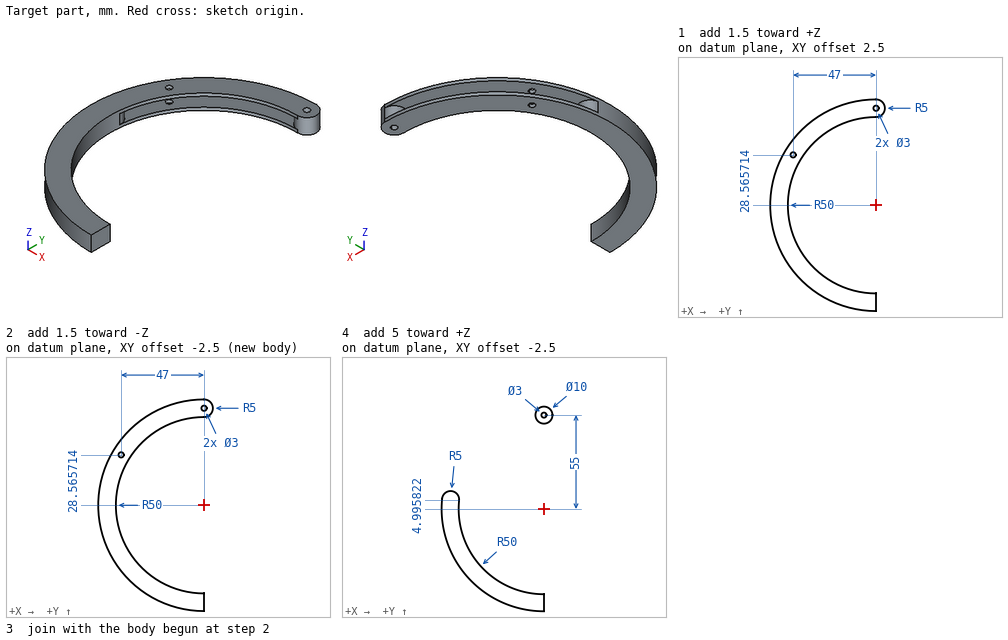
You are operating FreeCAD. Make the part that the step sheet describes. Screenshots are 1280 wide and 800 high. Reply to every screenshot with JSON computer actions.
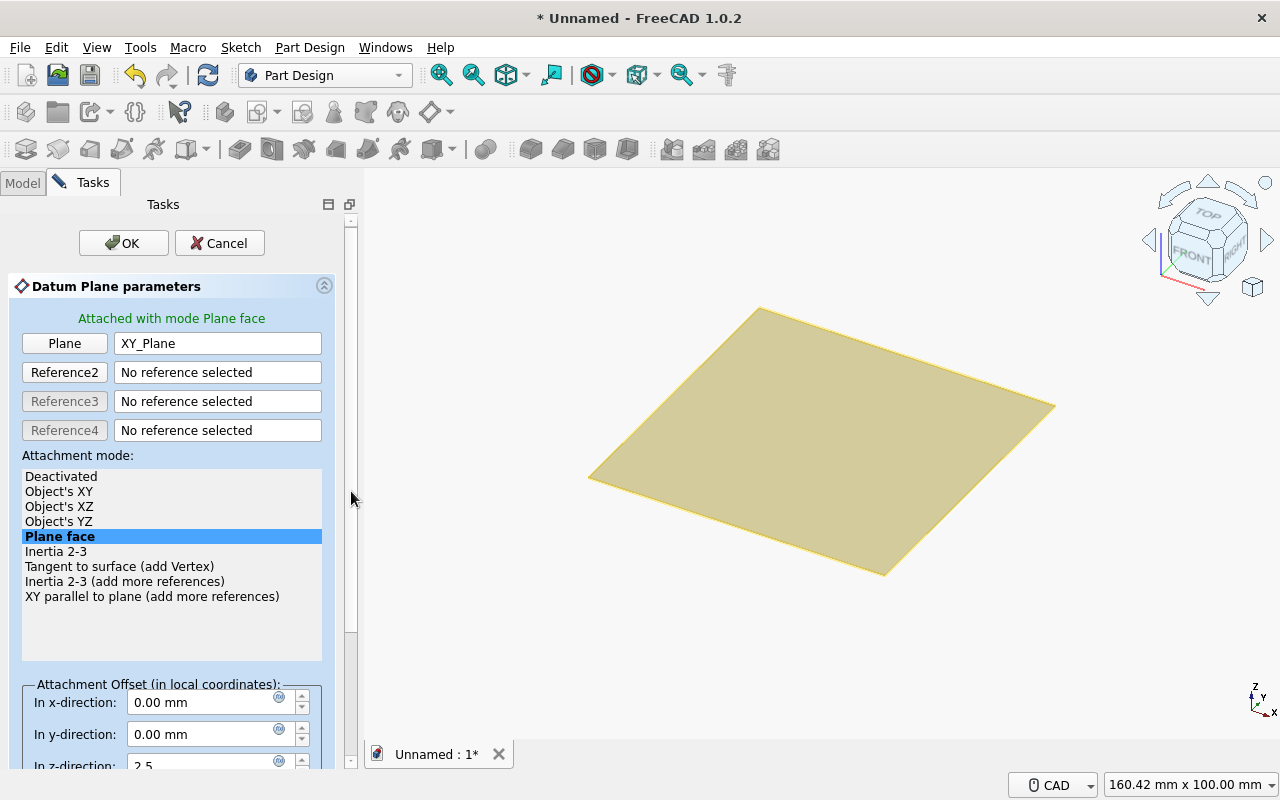
{"action": "left_click", "coordinate": [124, 243]}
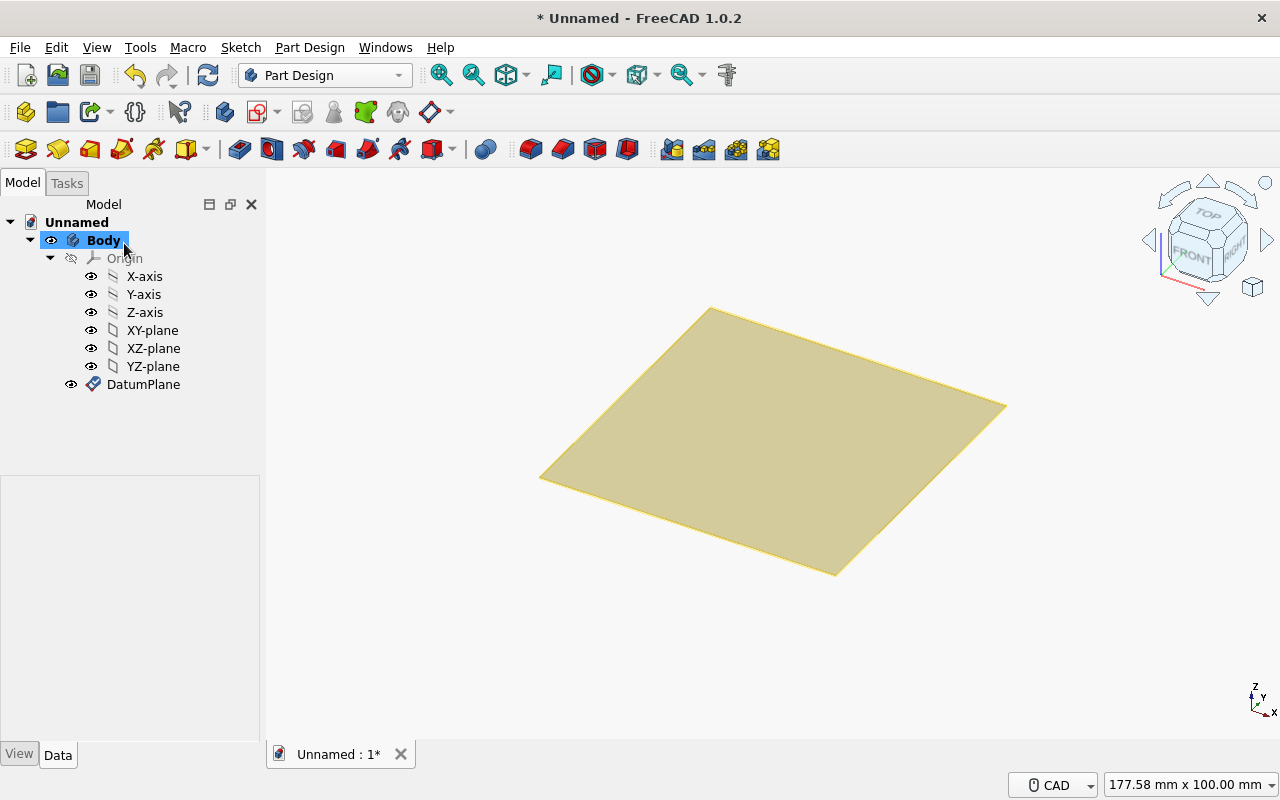
{"action": "left_click", "coordinate": [116, 384]}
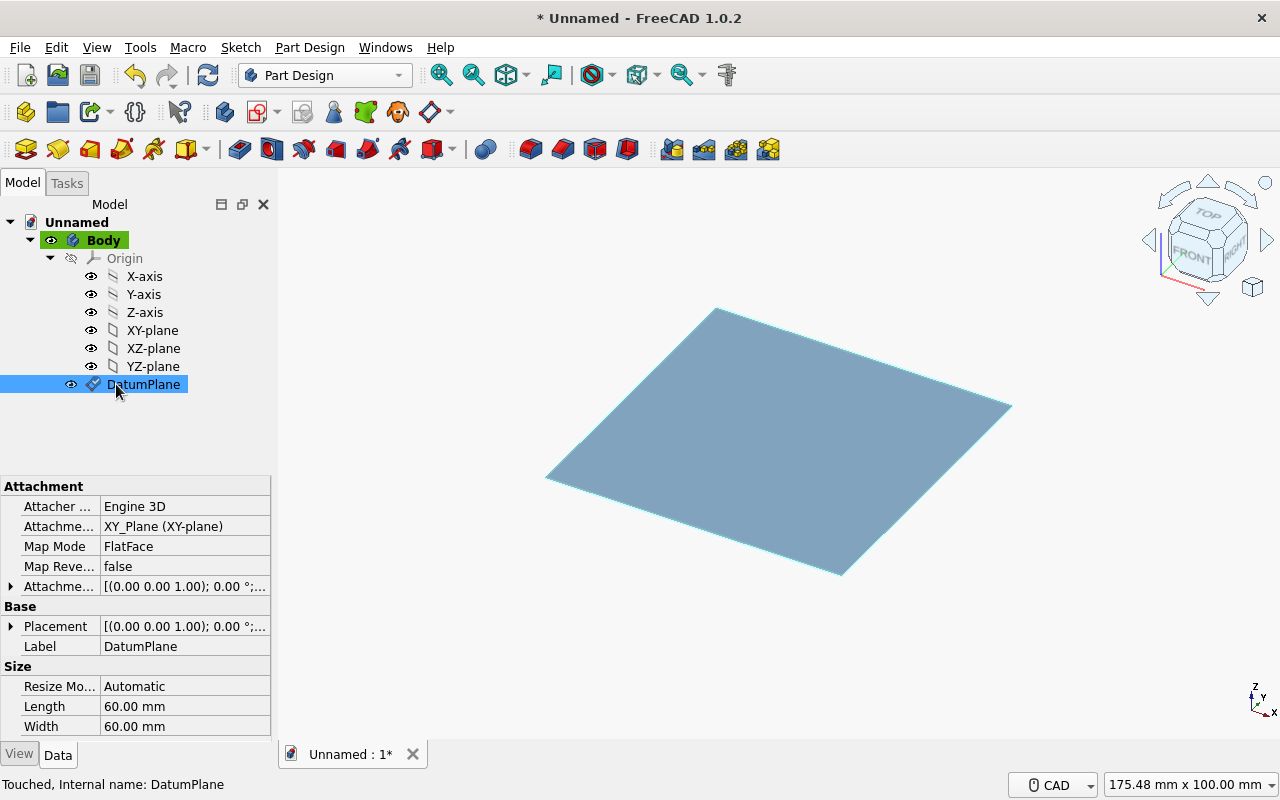
{"action": "left_click", "coordinate": [258, 112]}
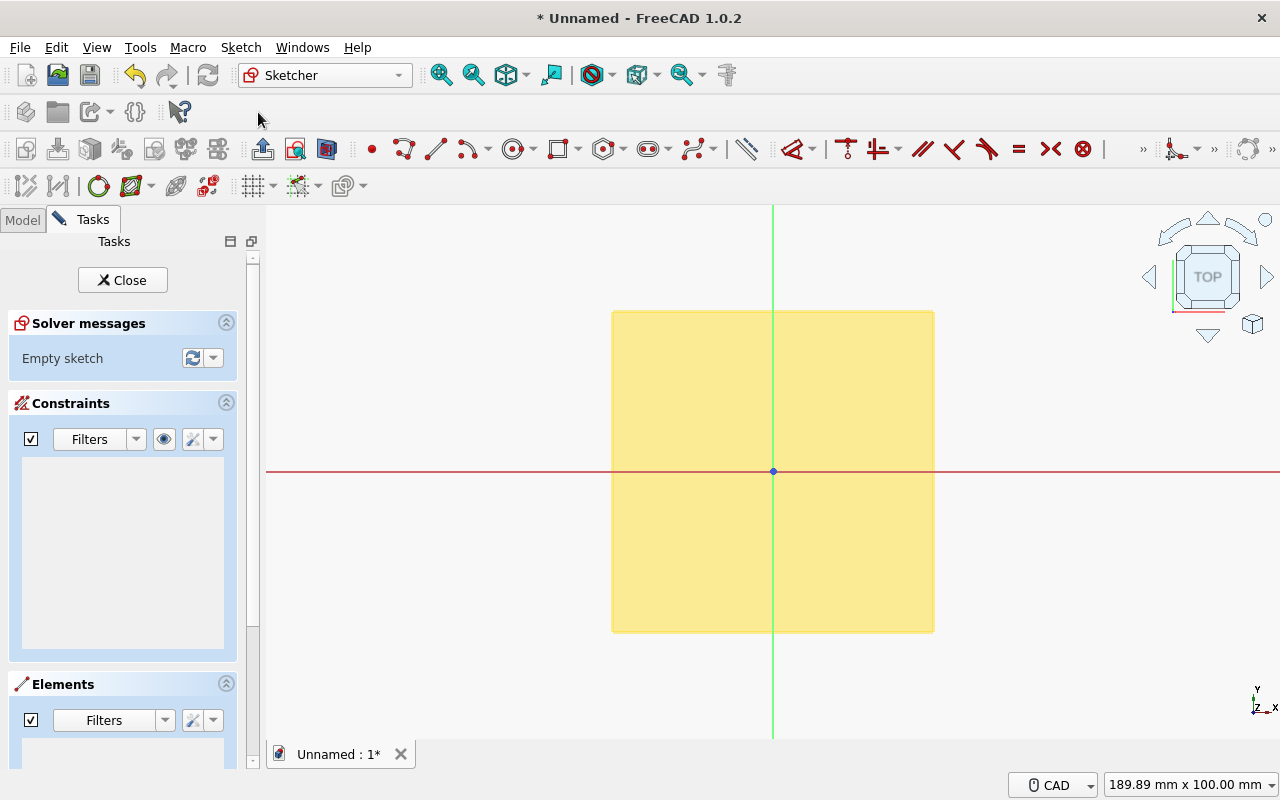
{"action": "scroll", "coordinate": [800, 472], "scroll_direction": "down", "scroll_amount": 3}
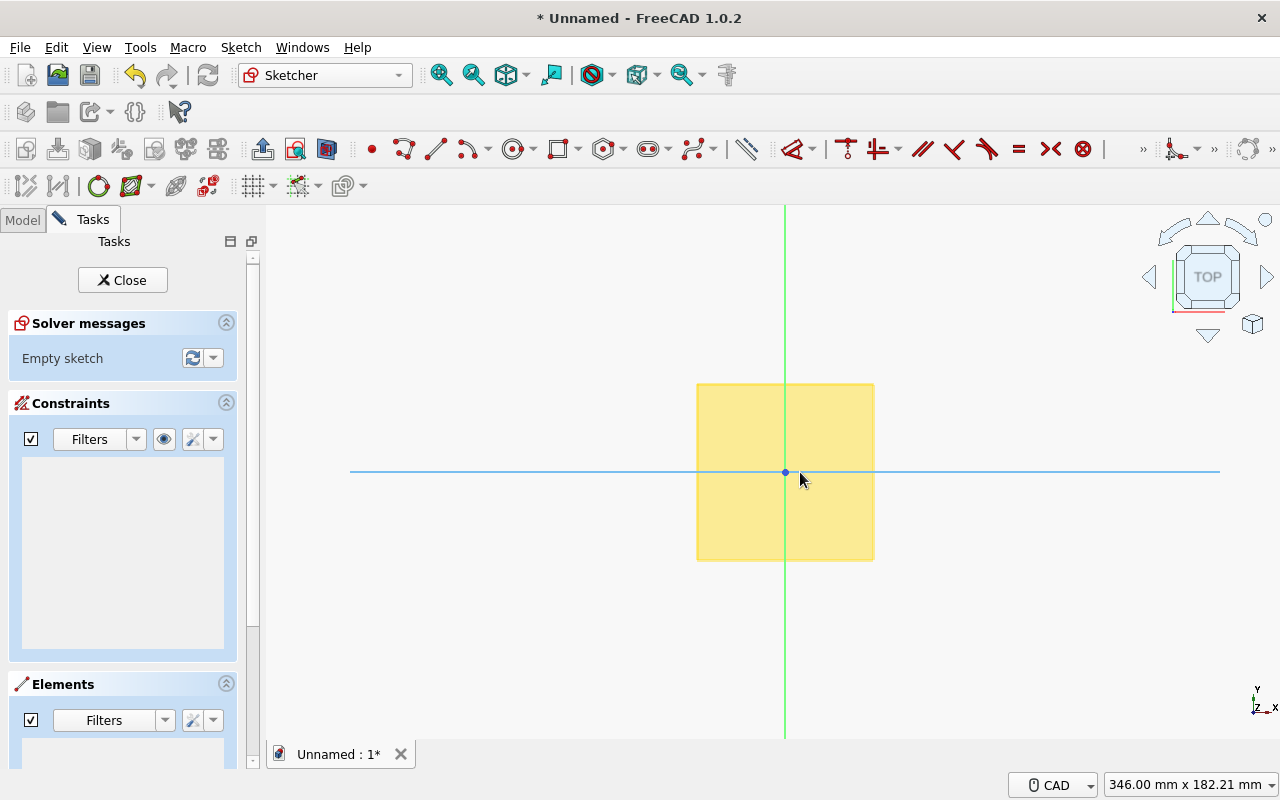
{"action": "left_click", "coordinate": [436, 150]}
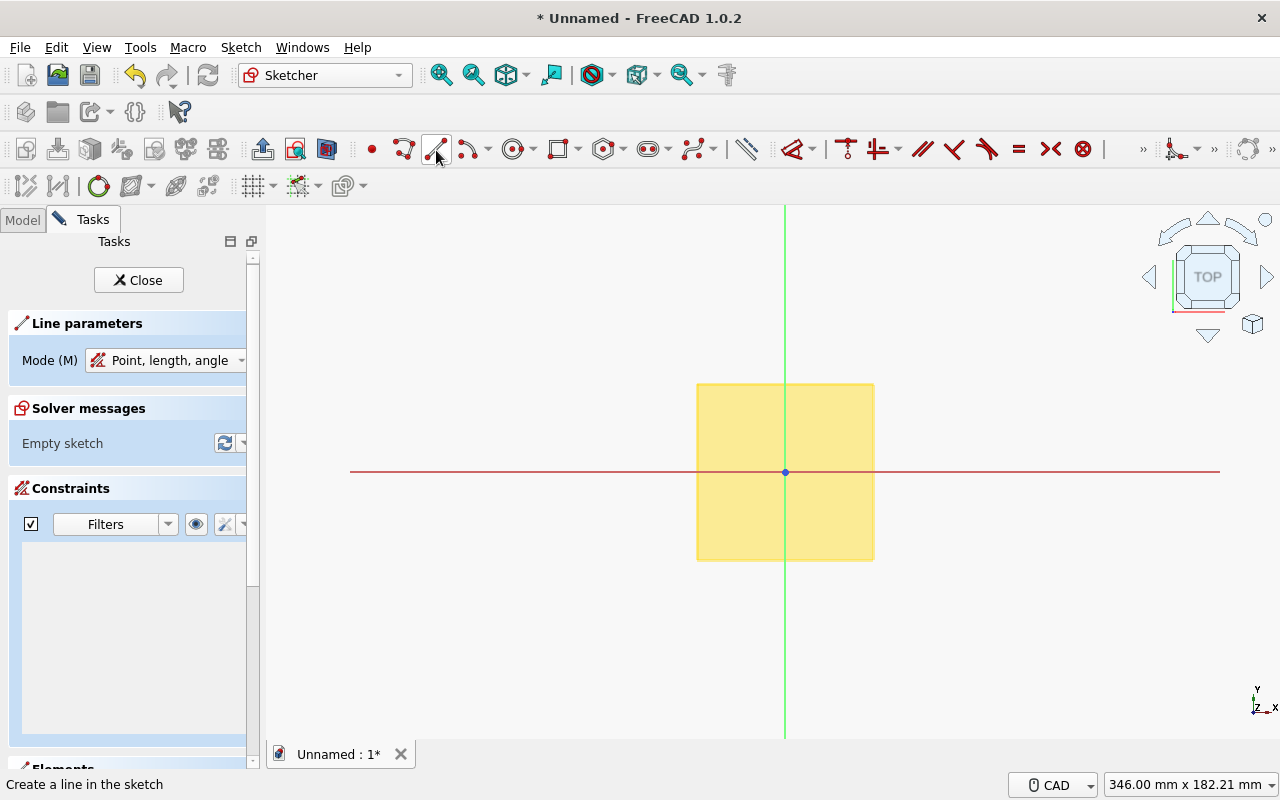
{"action": "left_click", "coordinate": [785, 648]}
{"action": "left_click", "coordinate": [776, 619]}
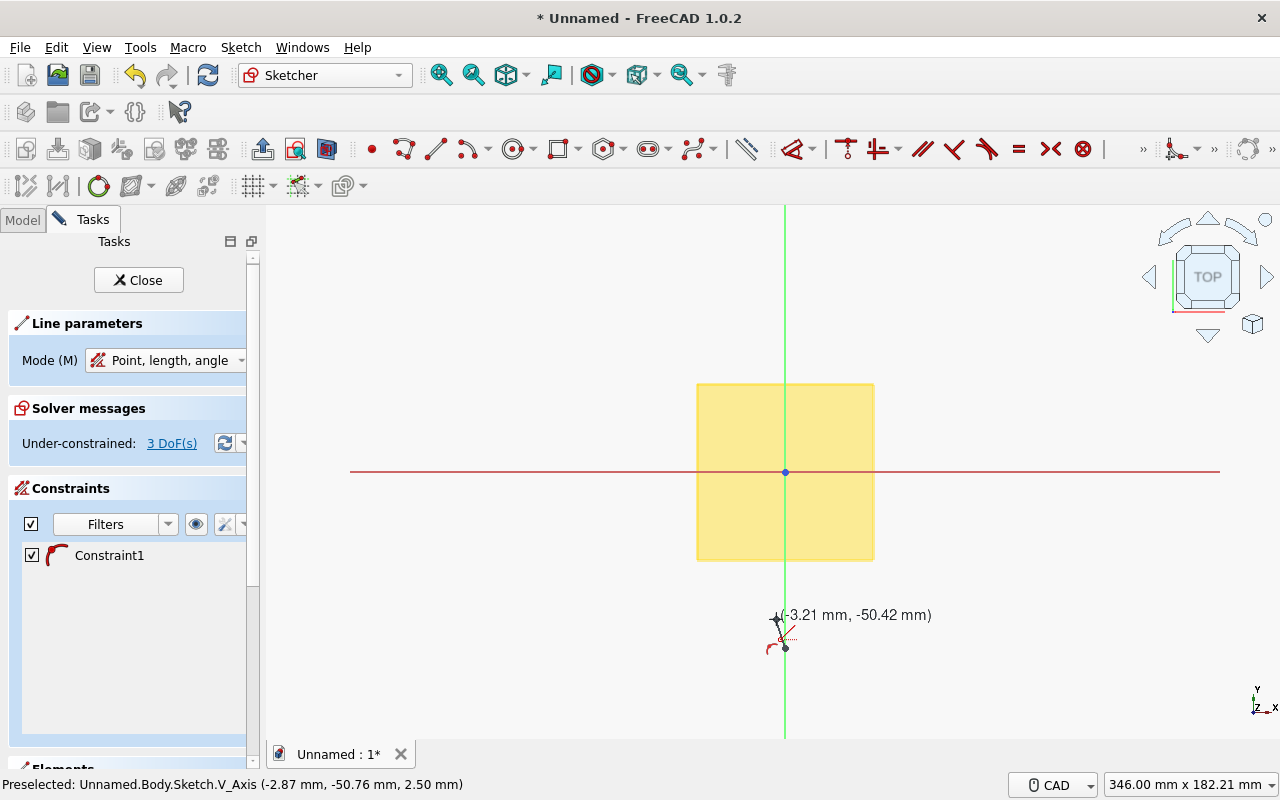
{"action": "key", "text": "g 3 a"}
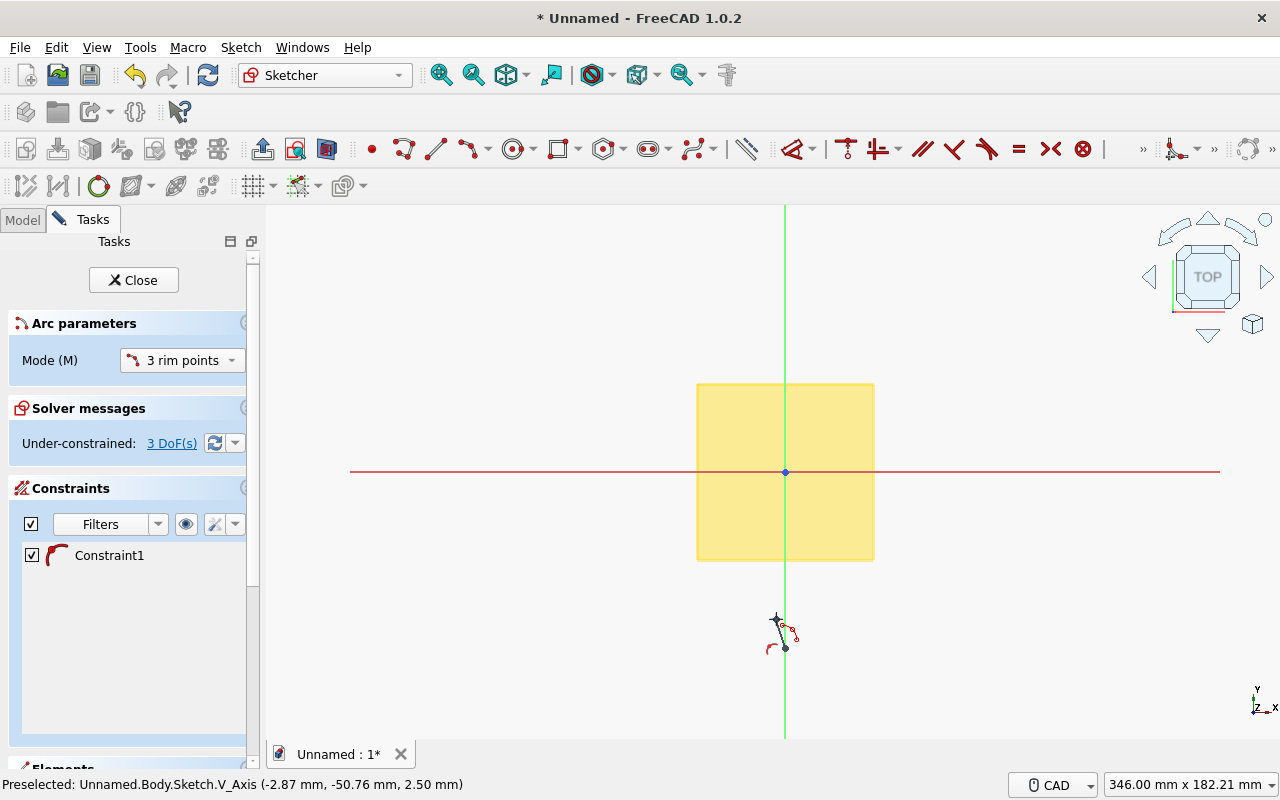
{"action": "left_click", "coordinate": [776, 620]}
{"action": "left_click", "coordinate": [785, 326]}
{"action": "left_click", "coordinate": [646, 427]}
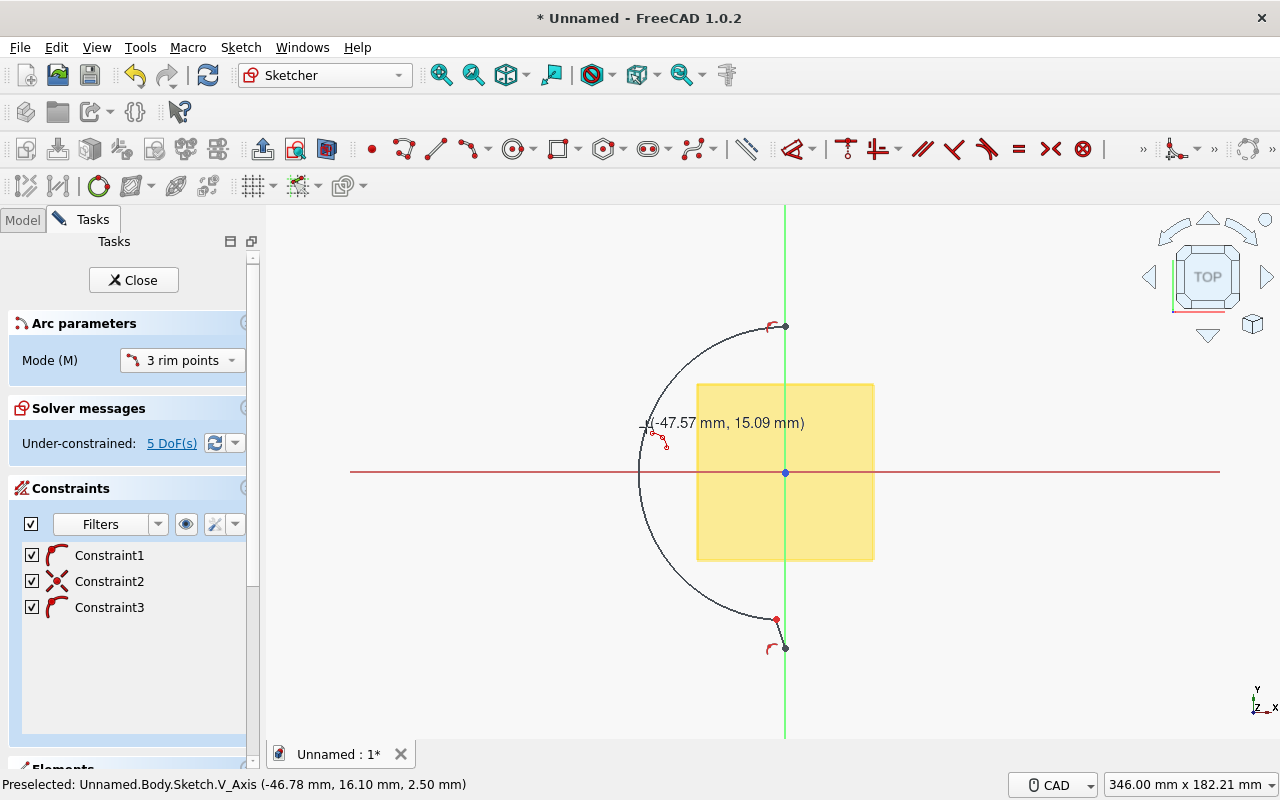
{"action": "left_click", "coordinate": [785, 327]}
{"action": "left_click", "coordinate": [785, 296]}
{"action": "left_click", "coordinate": [800, 311]}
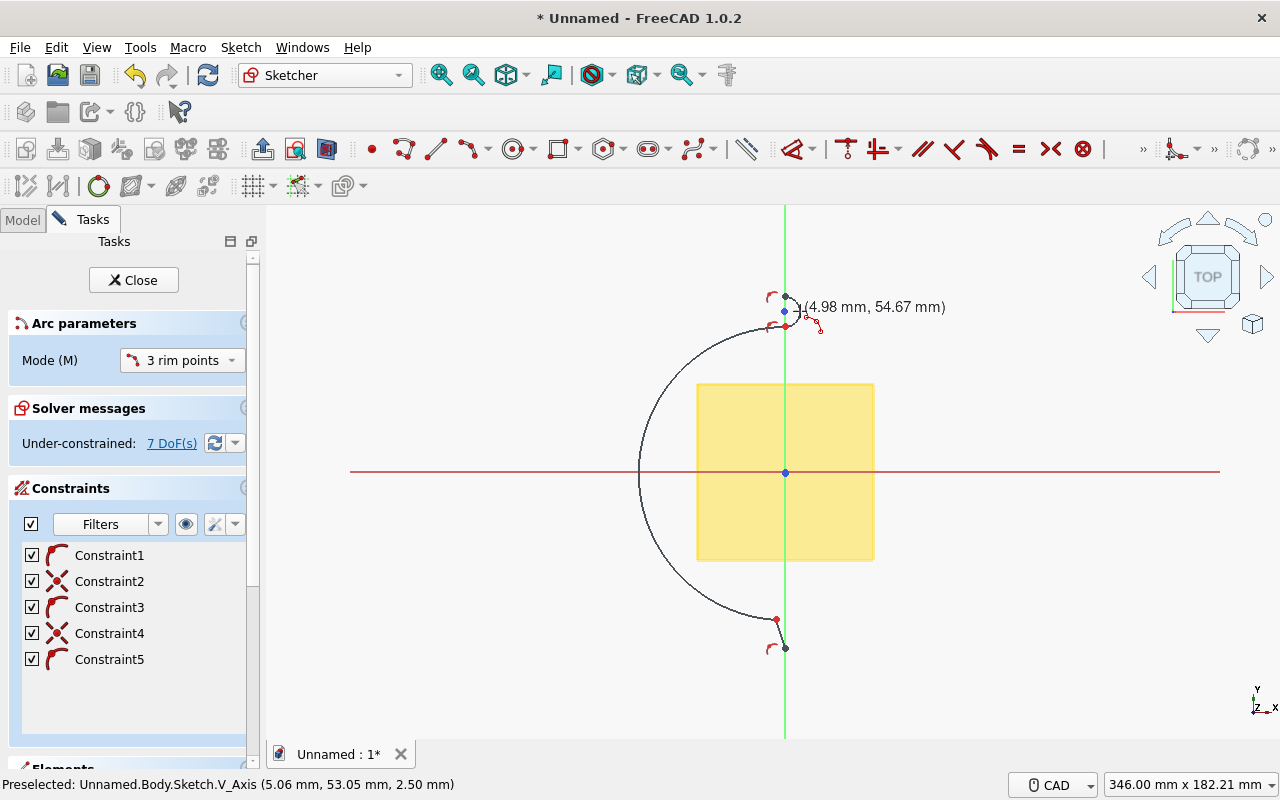
{"action": "left_click", "coordinate": [785, 297]}
{"action": "left_click", "coordinate": [785, 649]}
{"action": "left_click", "coordinate": [618, 418]}